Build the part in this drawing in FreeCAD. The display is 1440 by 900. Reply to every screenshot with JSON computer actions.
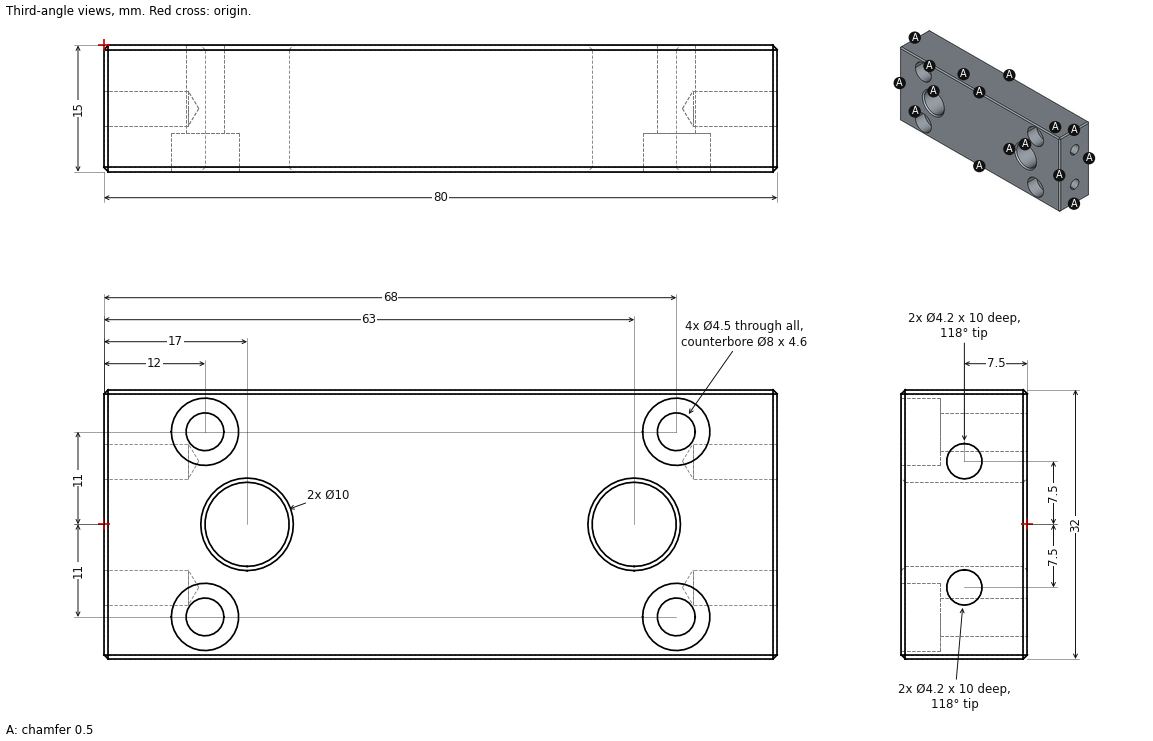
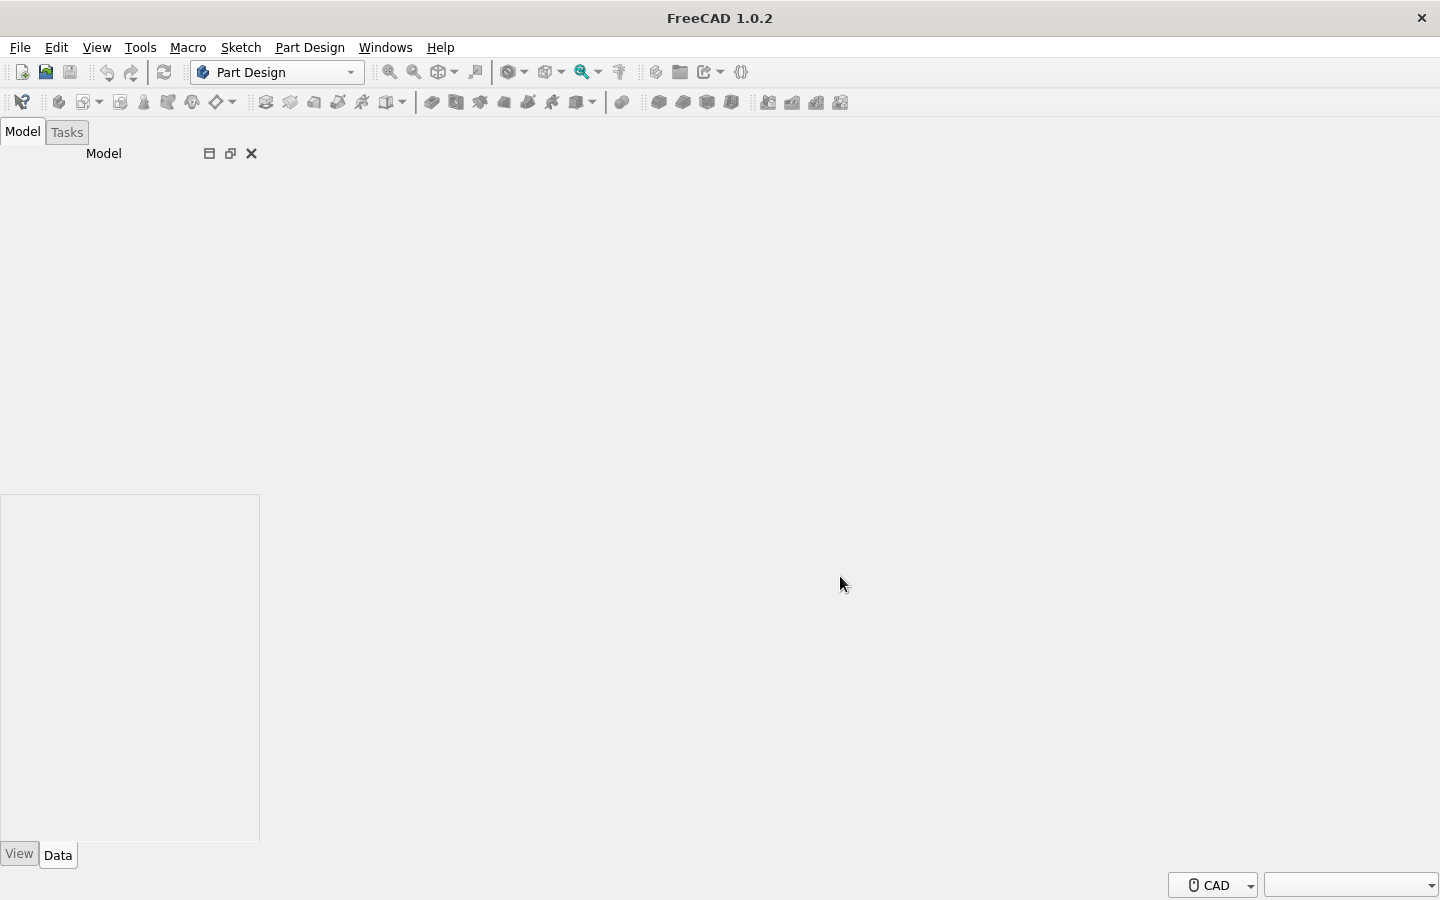
{"action": "left_click", "coordinate": [22, 72]}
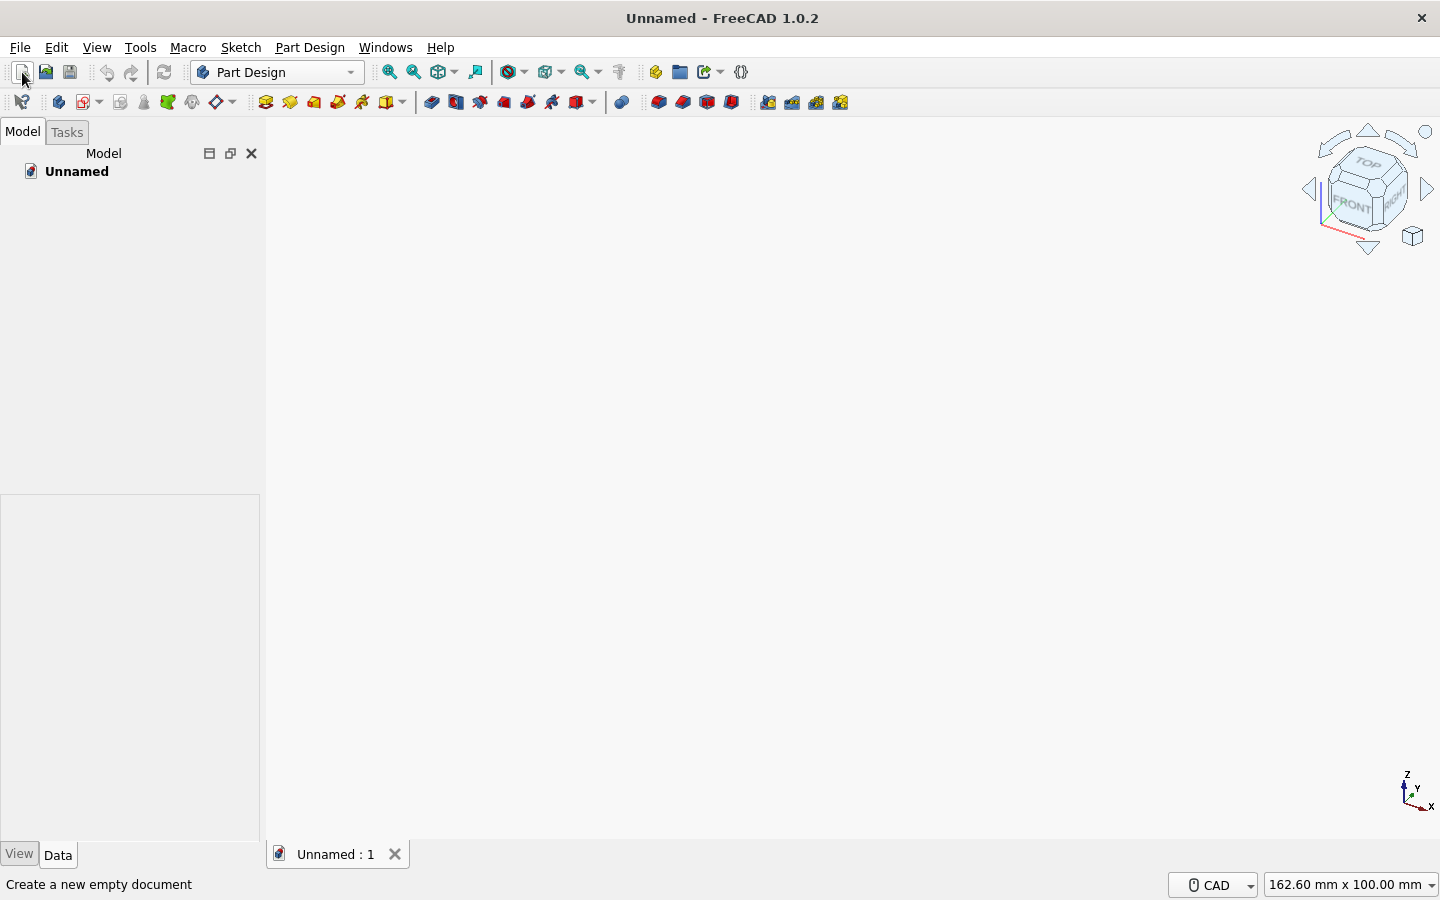
{"action": "left_click", "coordinate": [84, 102]}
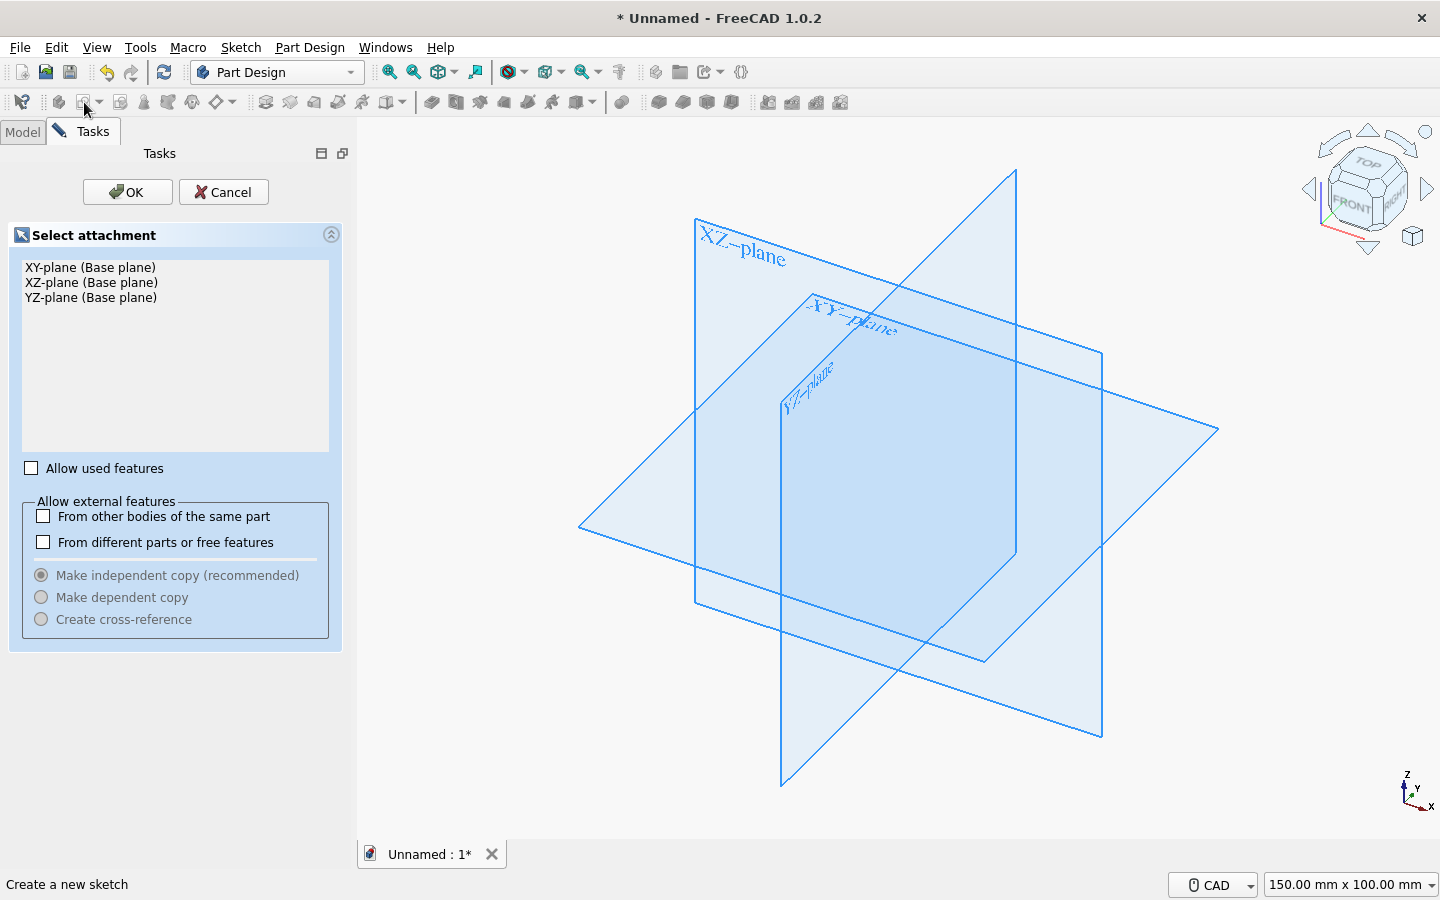
{"action": "left_click", "coordinate": [82, 268]}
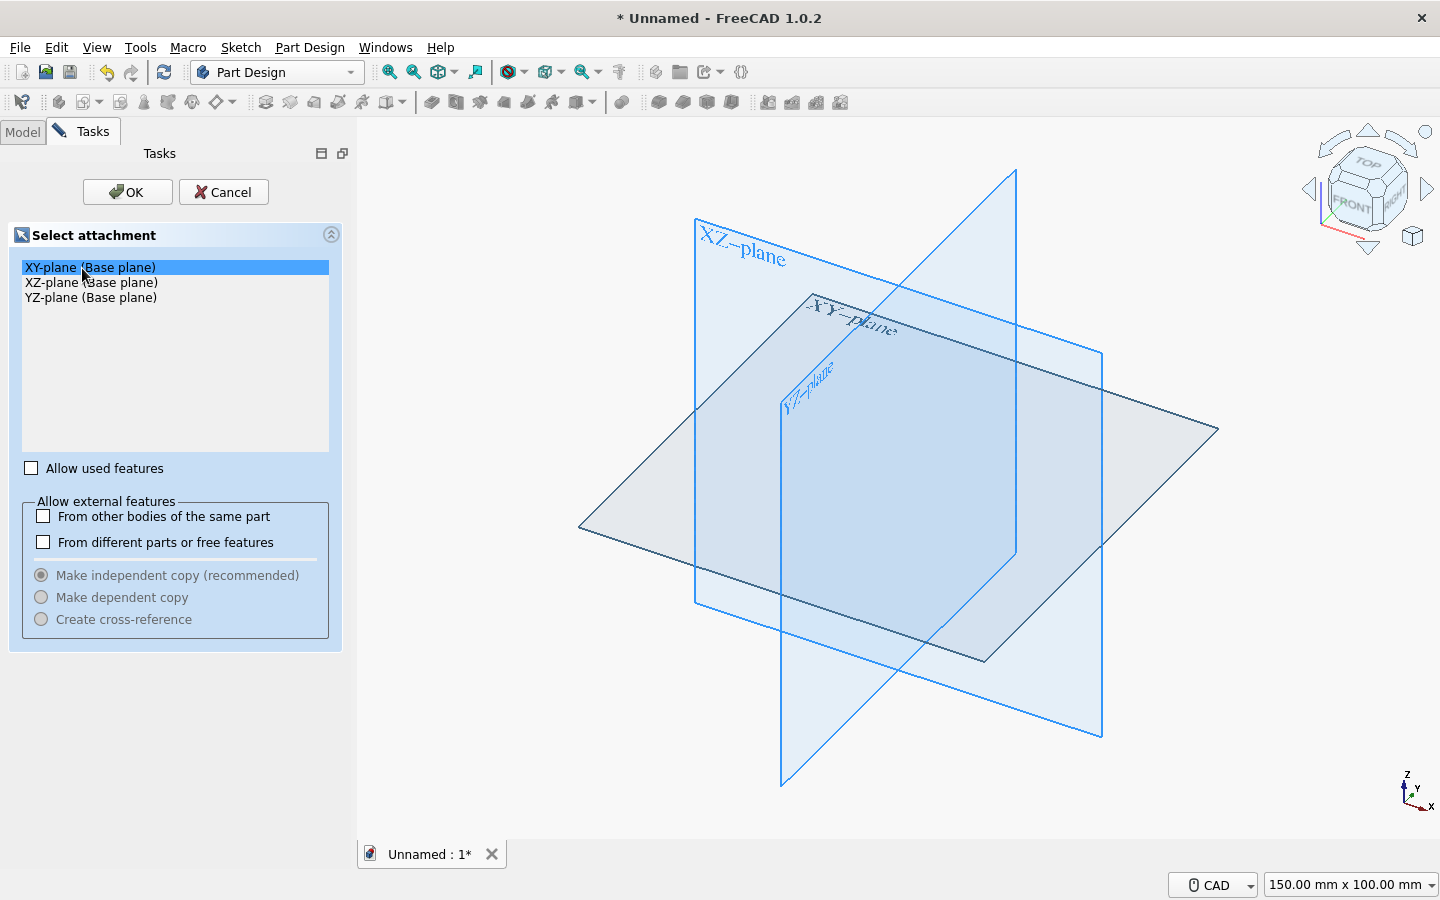
{"action": "left_click", "coordinate": [128, 192]}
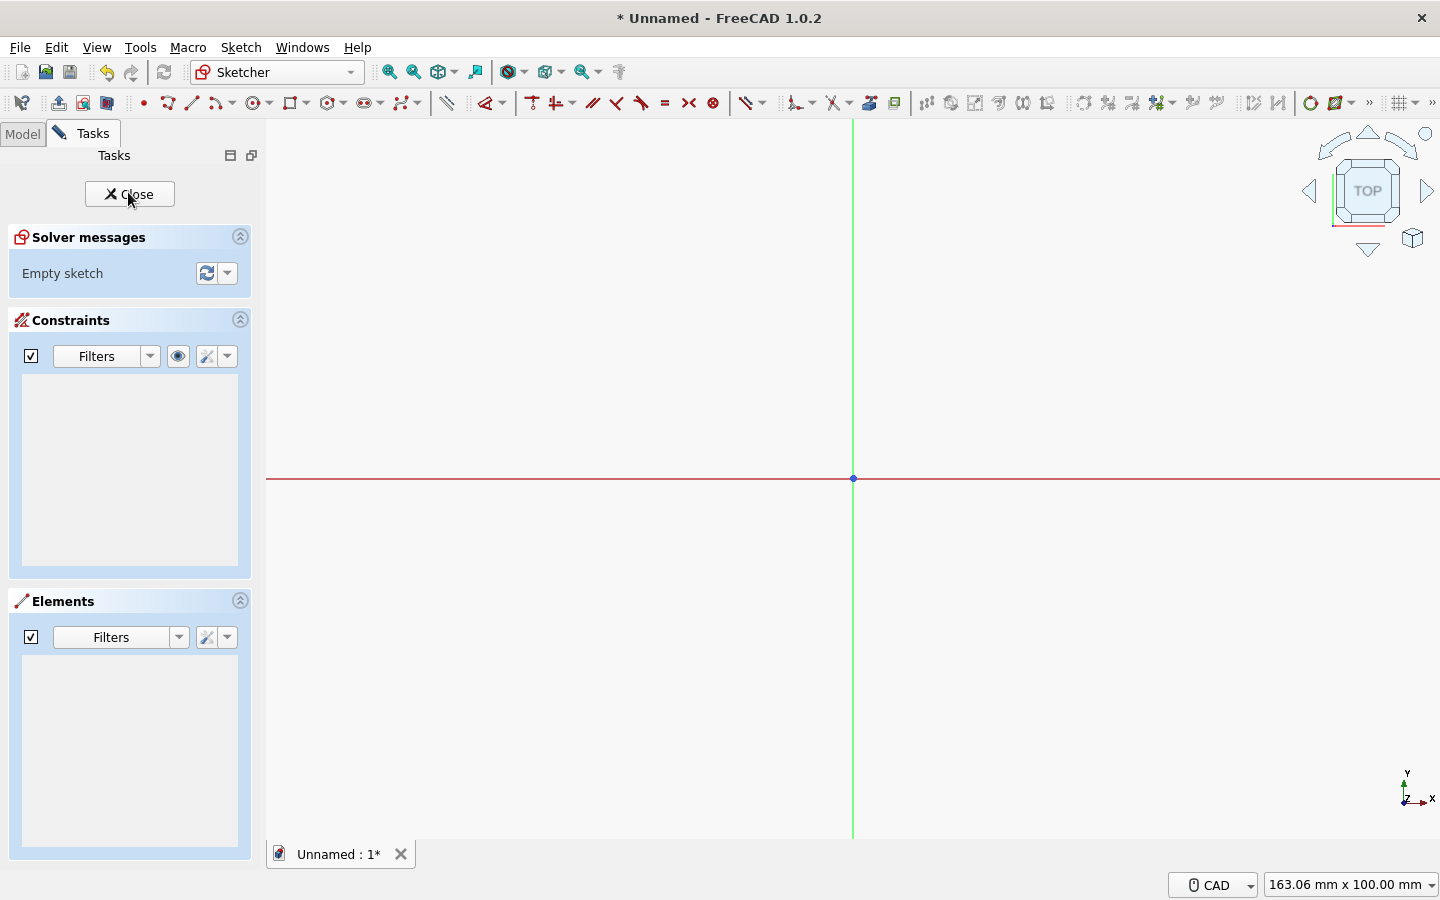
{"action": "scroll", "coordinate": [294, 235], "scroll_direction": "down", "scroll_amount": 1}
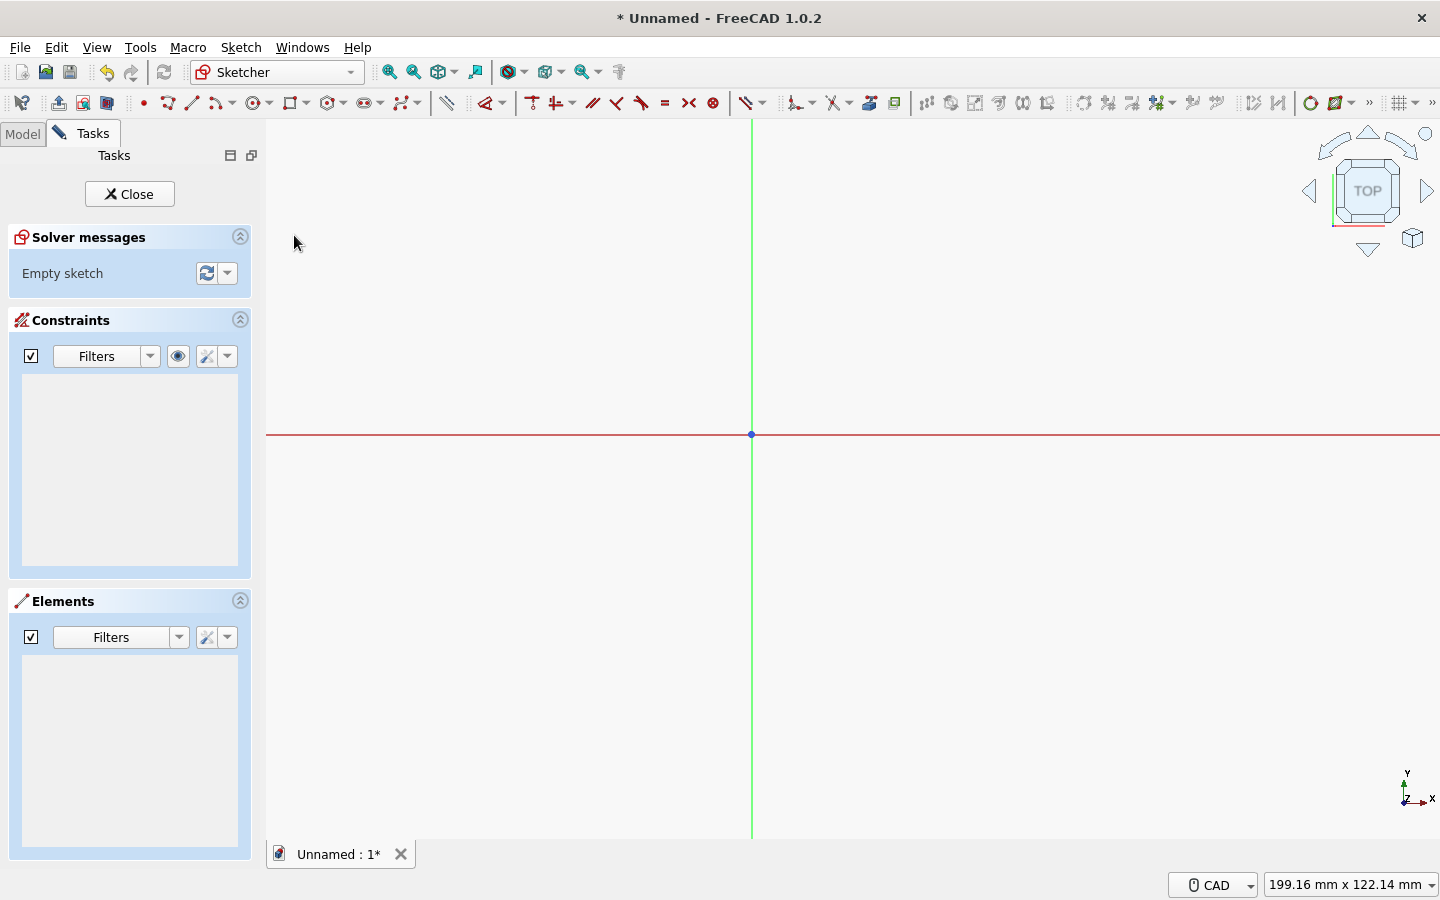
{"action": "scroll", "coordinate": [1275, 479], "scroll_direction": "up", "scroll_amount": 2}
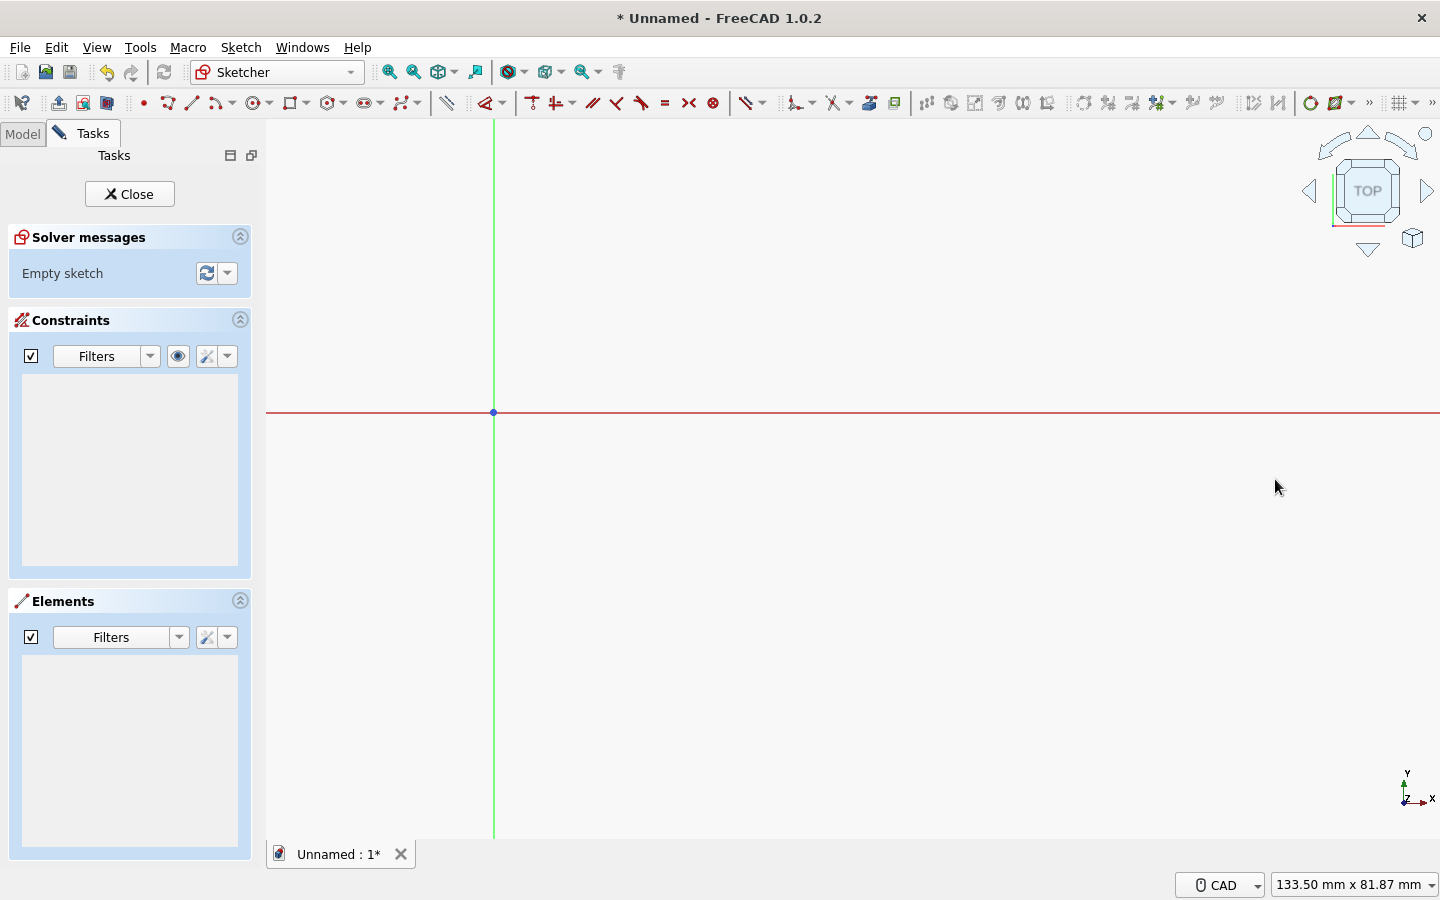
{"action": "left_click", "coordinate": [290, 104]}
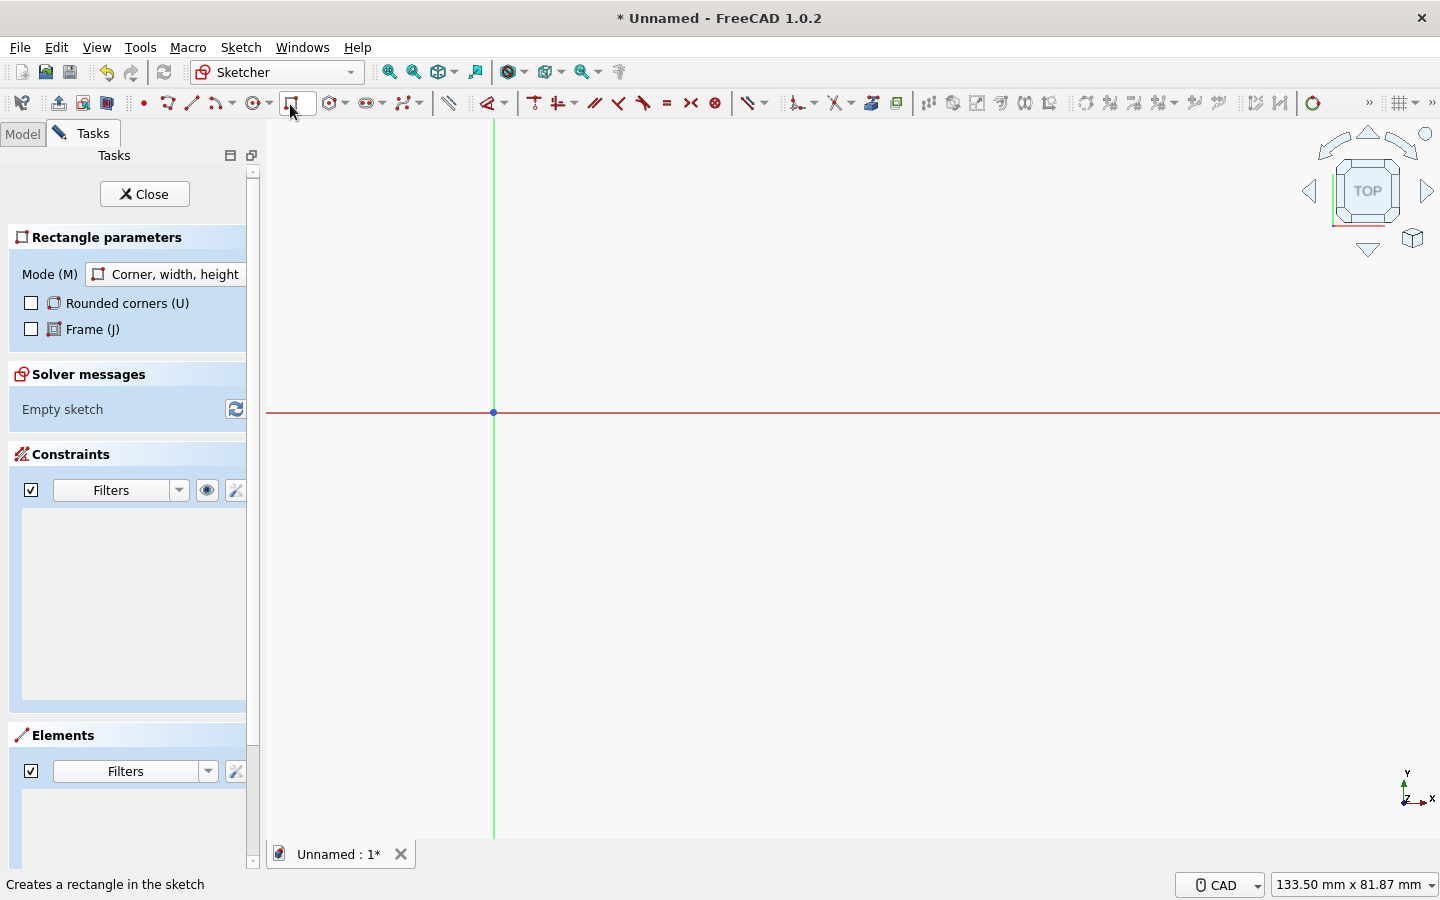
{"action": "left_click", "coordinate": [494, 413]}
{"action": "left_click", "coordinate": [1197, 545]}
{"action": "key", "text": "Escape"}